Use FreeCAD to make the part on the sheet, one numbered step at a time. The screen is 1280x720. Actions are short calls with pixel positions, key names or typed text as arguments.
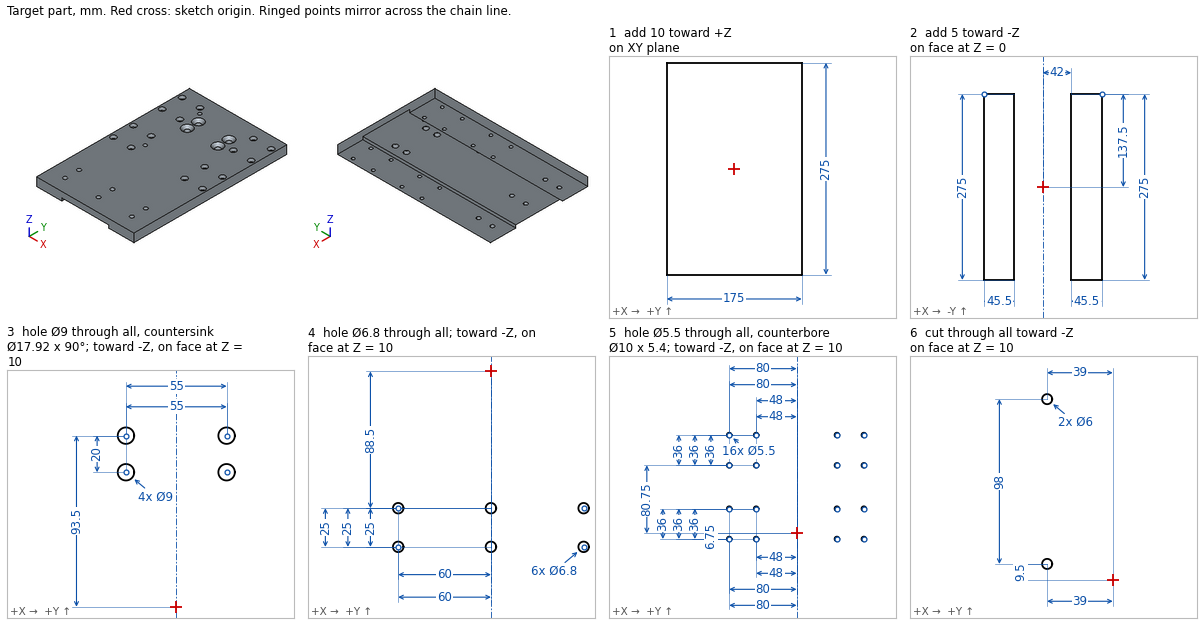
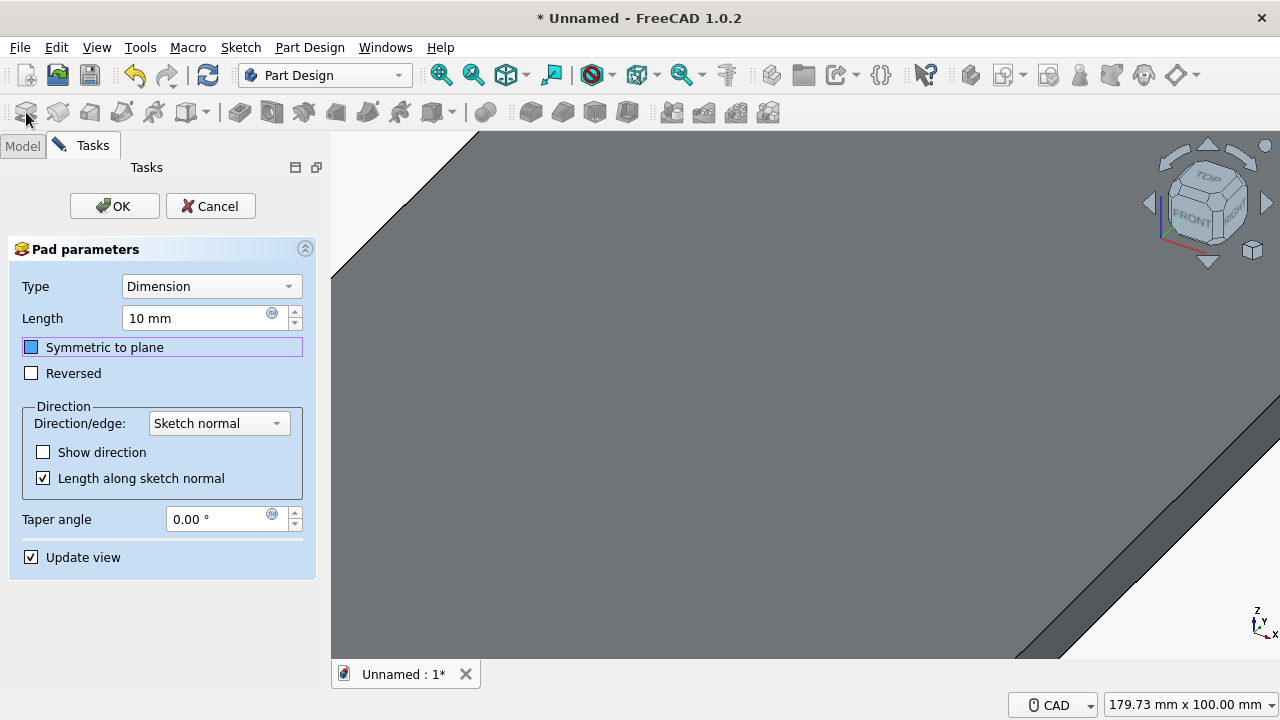
click(115, 206)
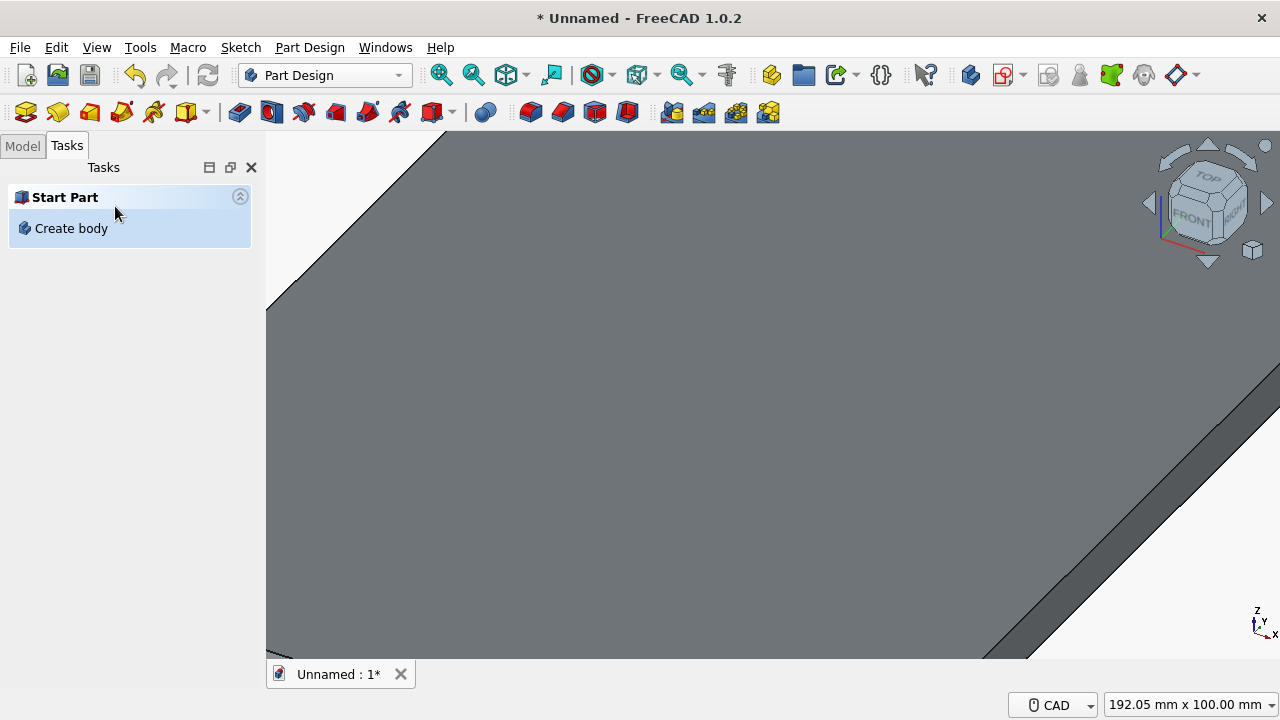
click(442, 76)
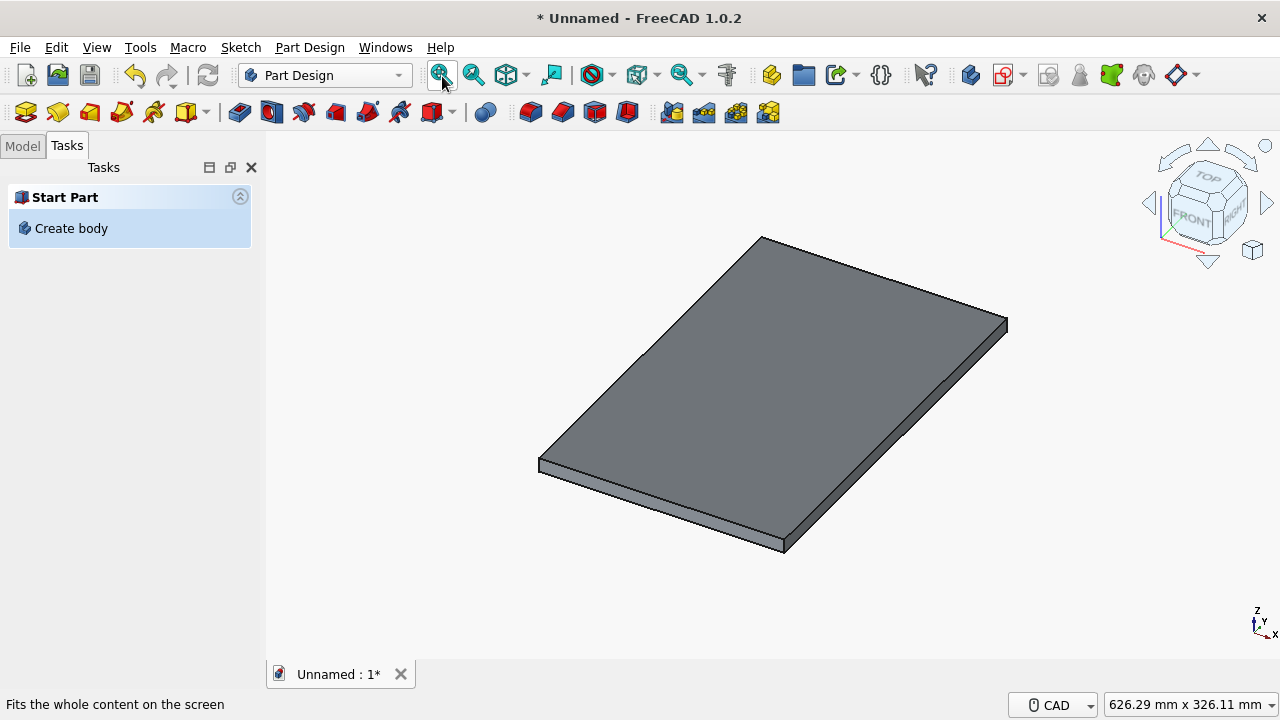
key(5)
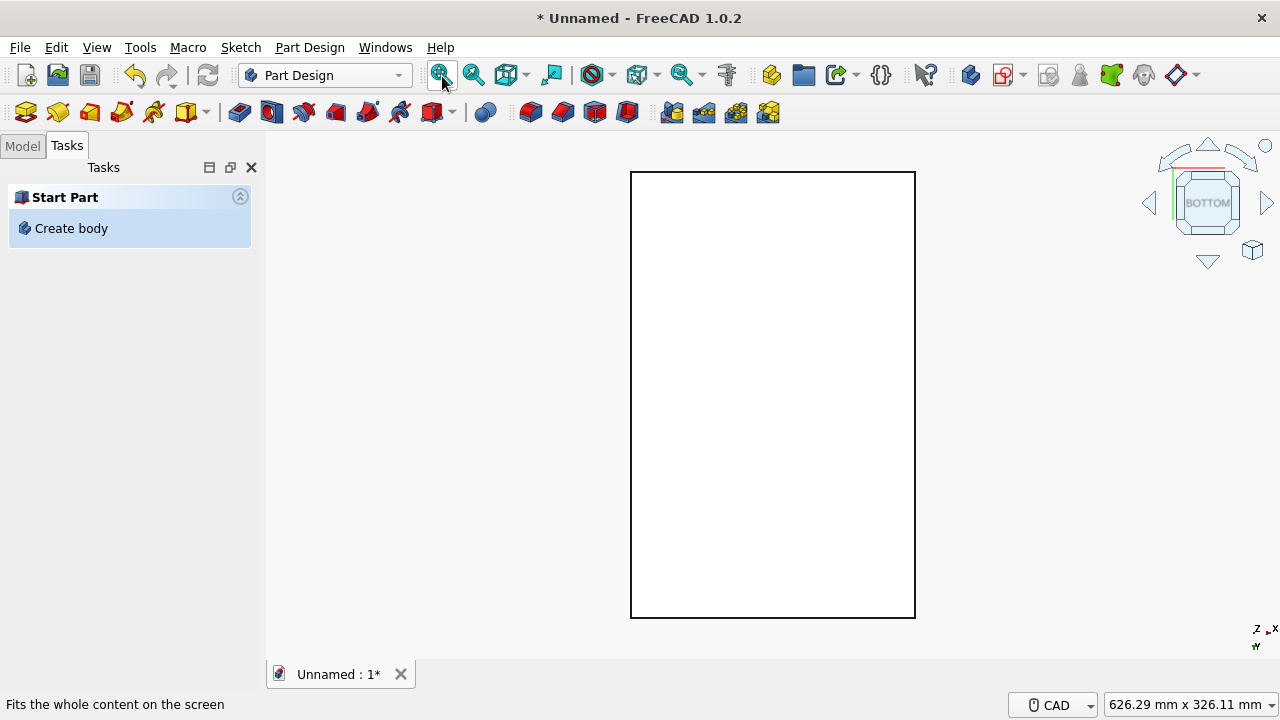
click(773, 458)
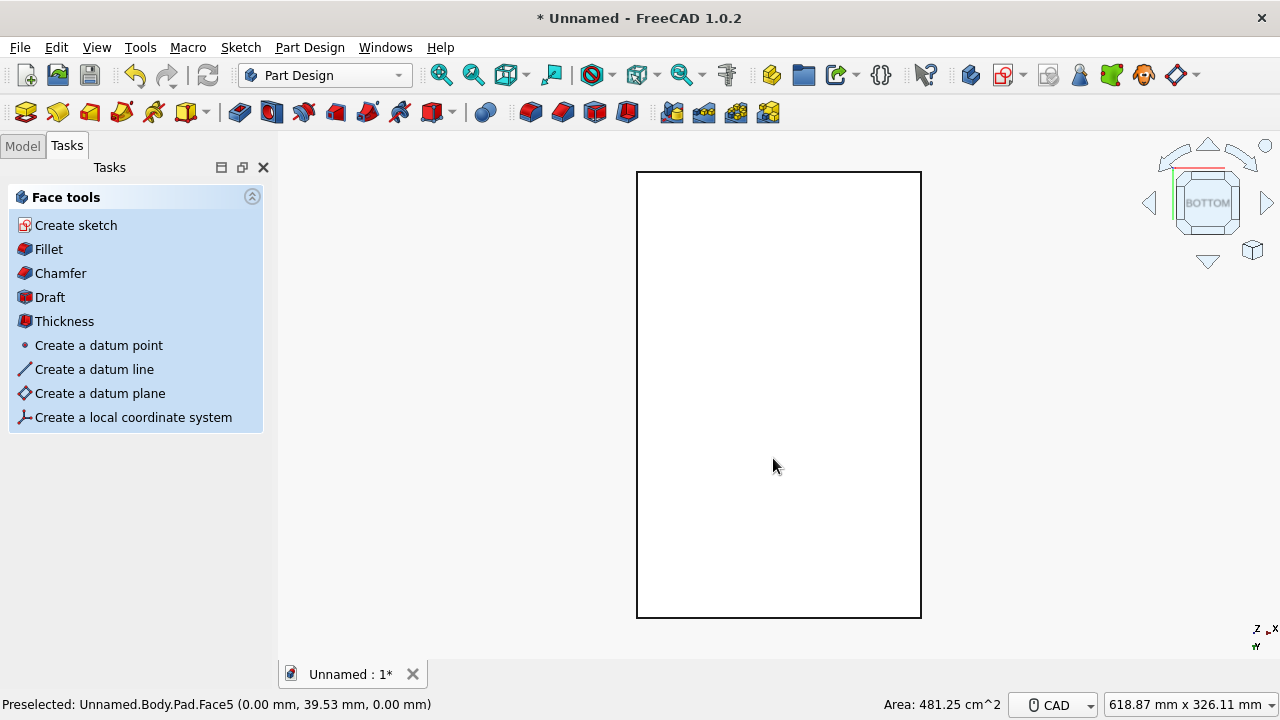
click(1004, 76)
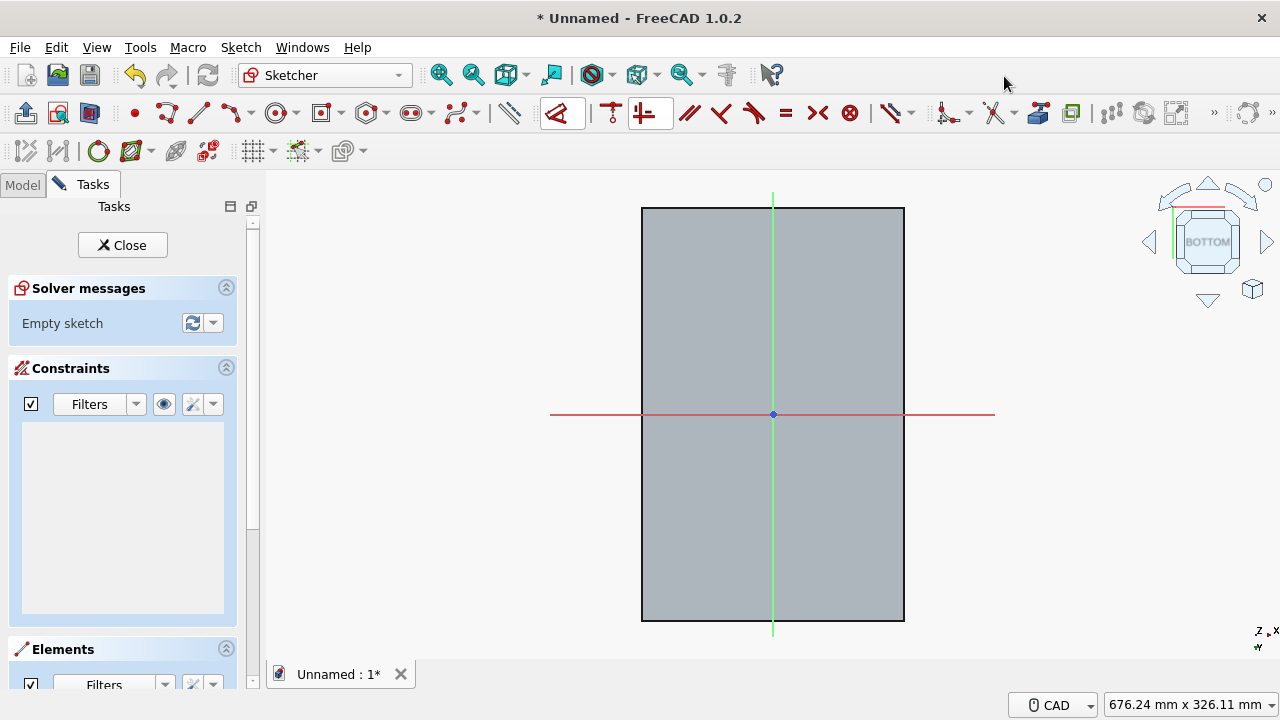
scroll(395, 415, down, 1)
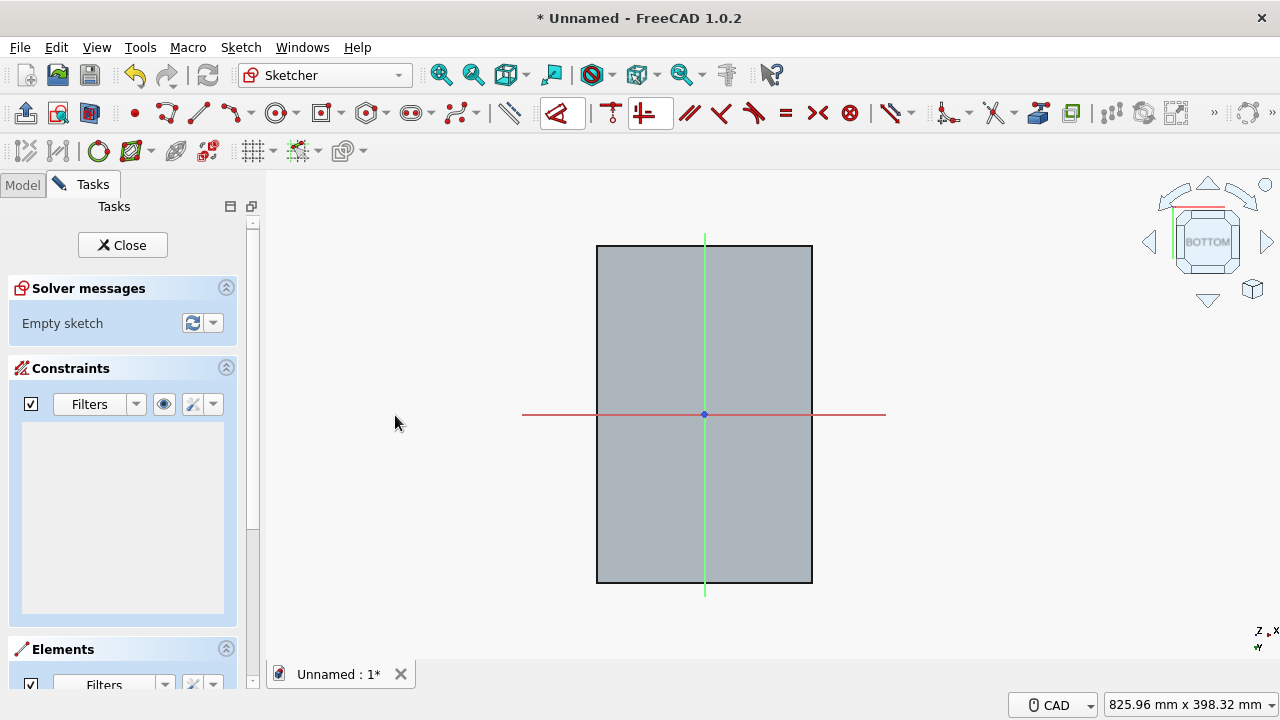
key(g)
key(r)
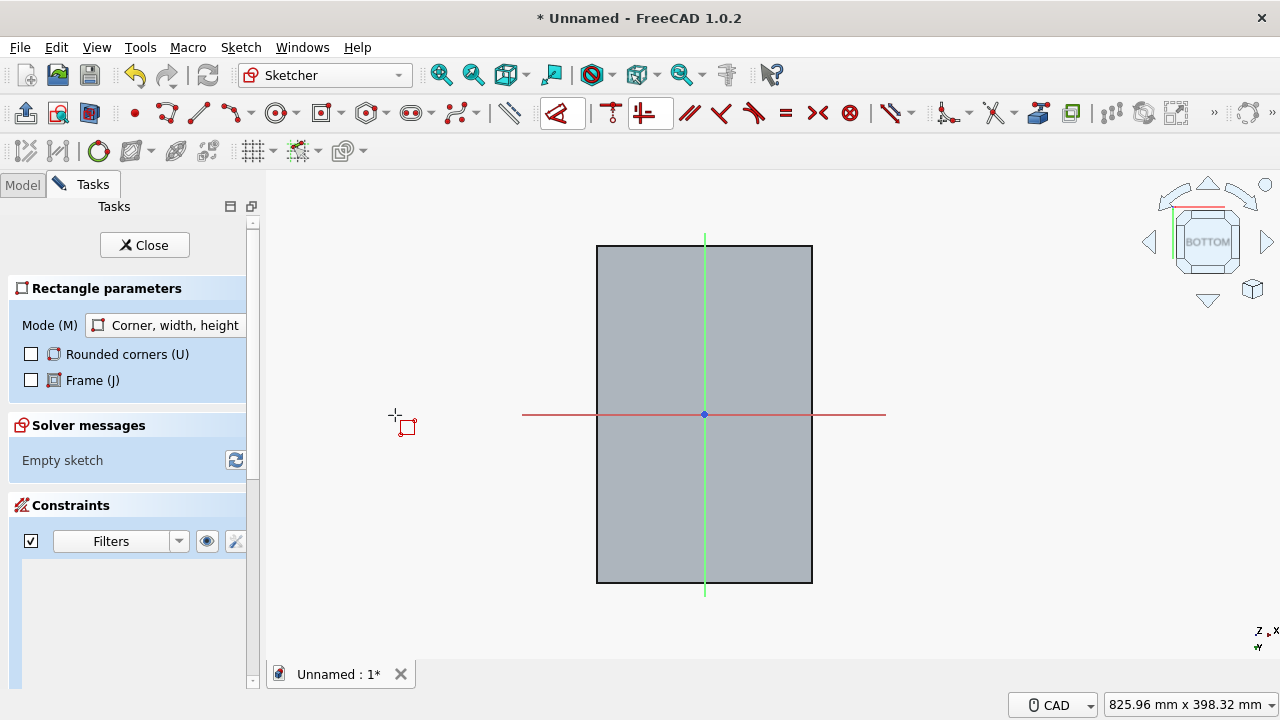
click(756, 246)
move(812, 583)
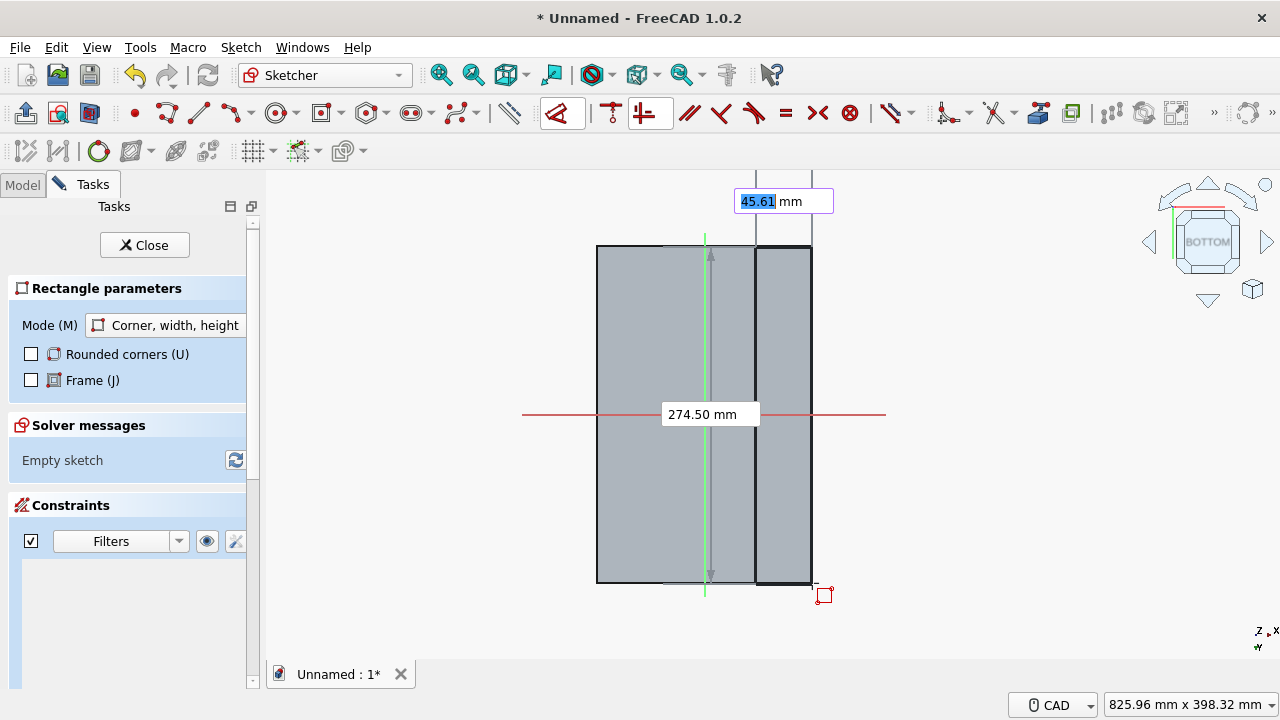
text(45.5)
key(Tab)
text(275)
key(Return)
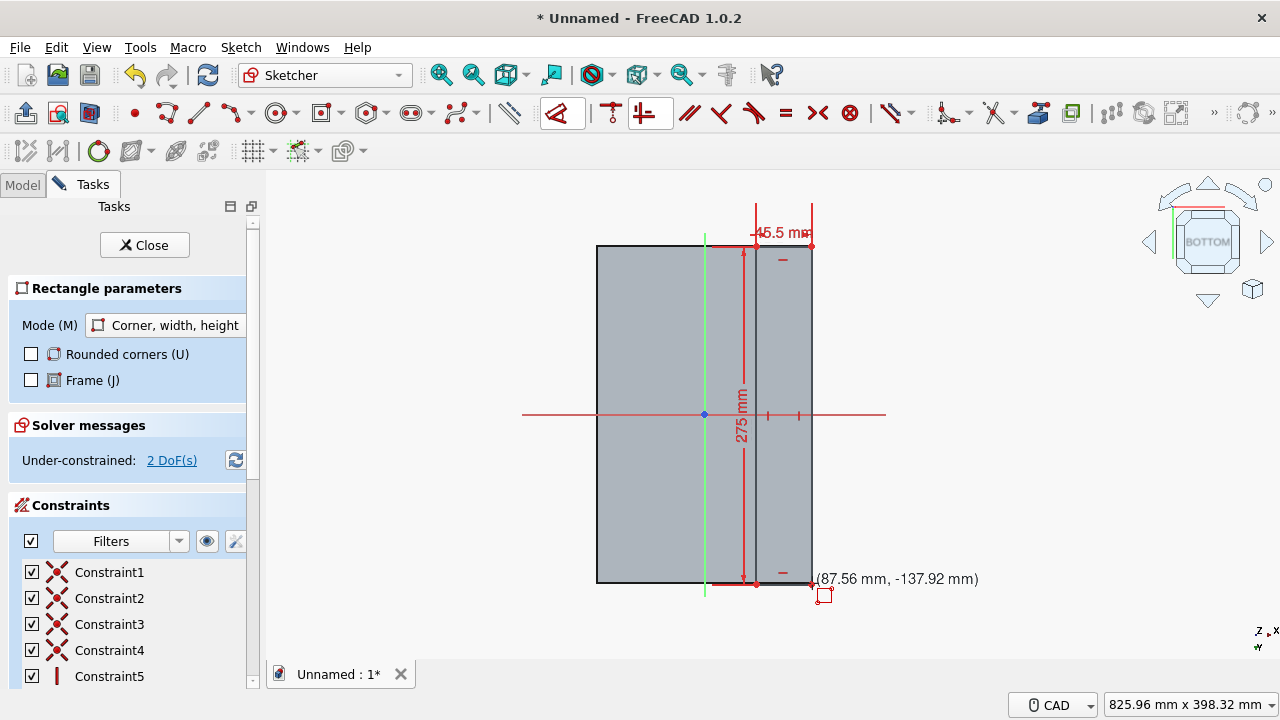
click(597, 246)
move(653, 583)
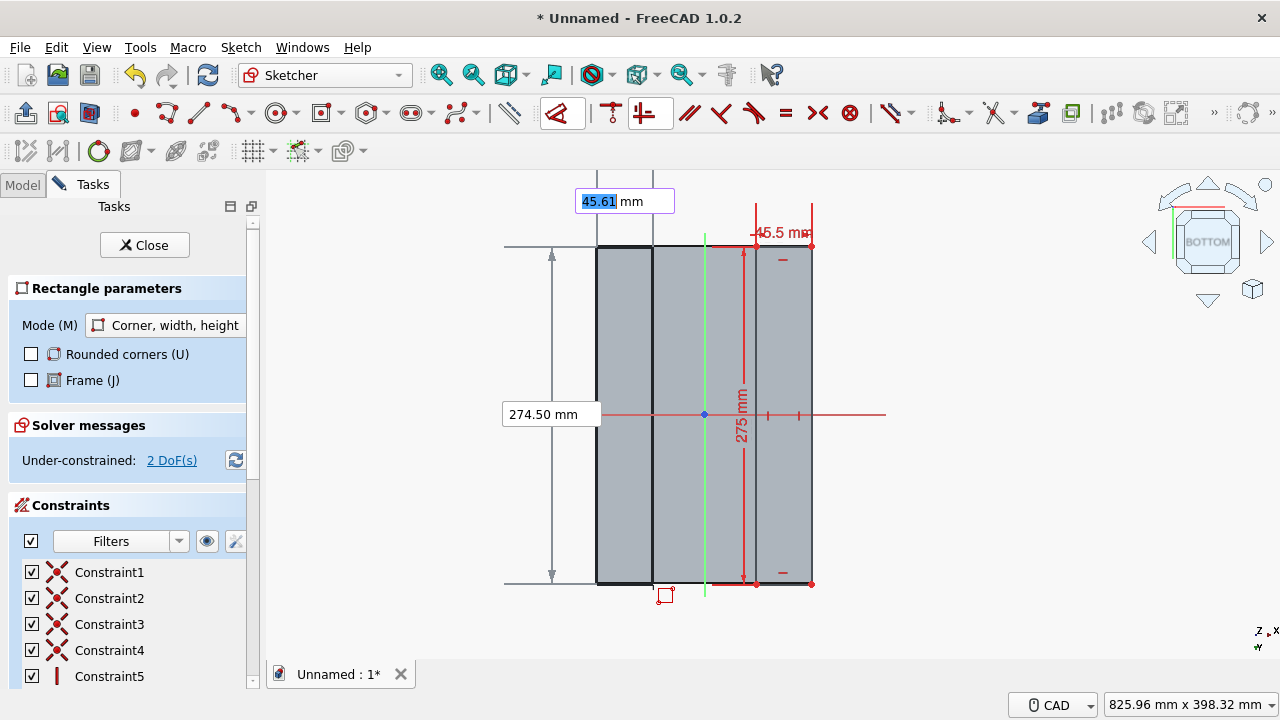
text(45.5)
key(Tab)
text(275)
key(Return)
key(Escape)